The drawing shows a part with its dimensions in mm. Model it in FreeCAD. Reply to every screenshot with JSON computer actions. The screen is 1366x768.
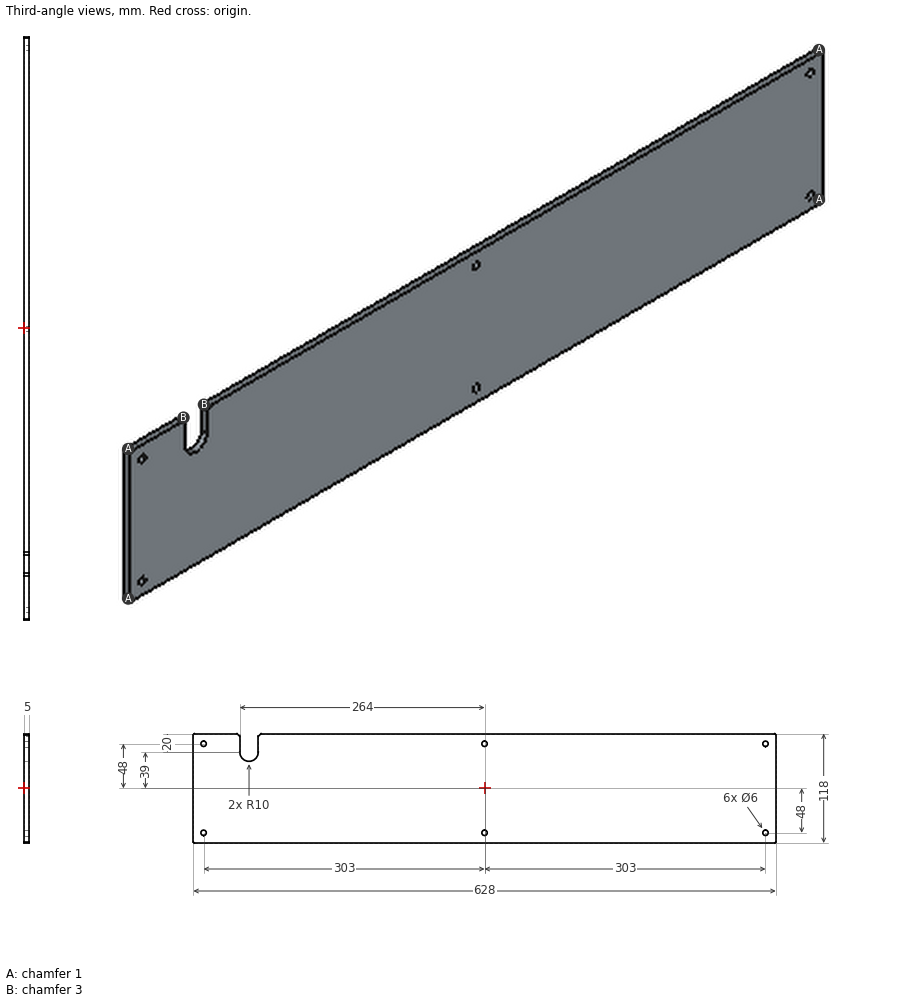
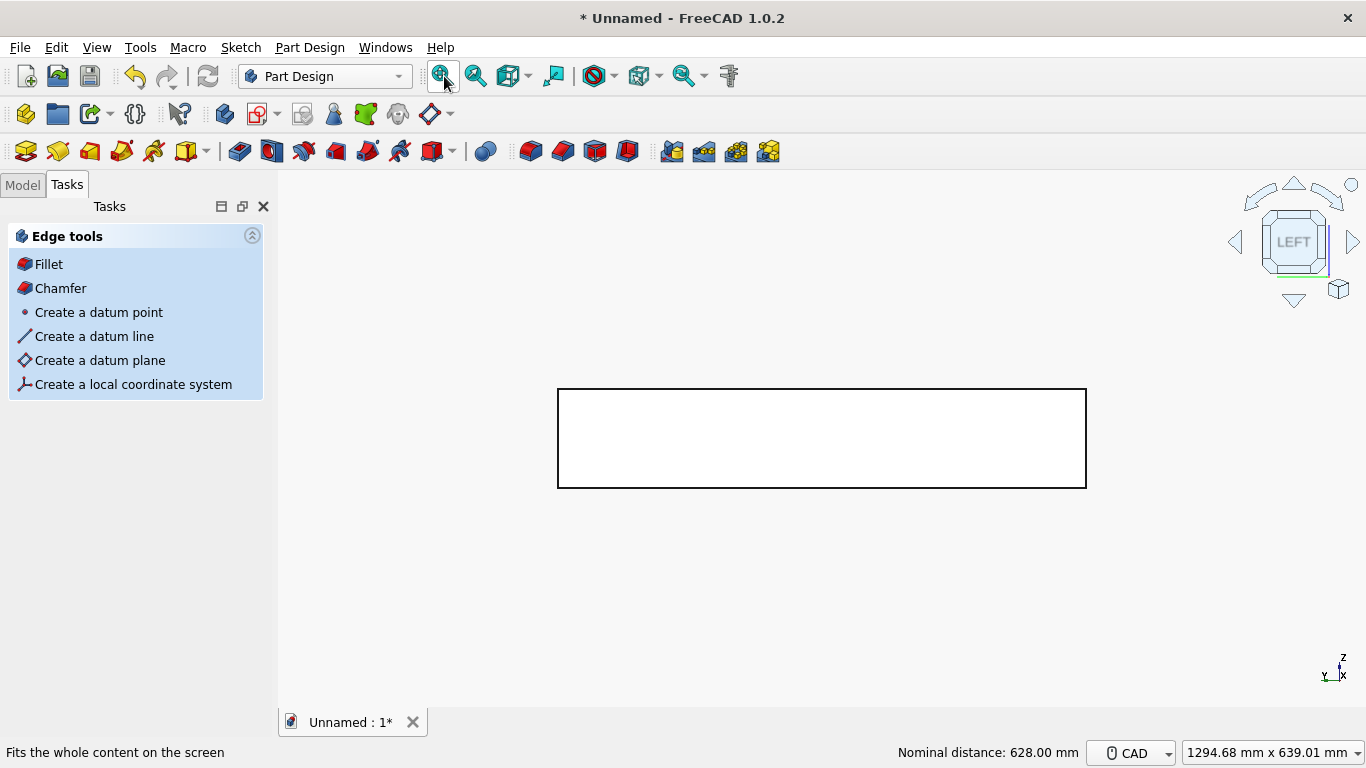
{"action": "key", "text": "v 3"}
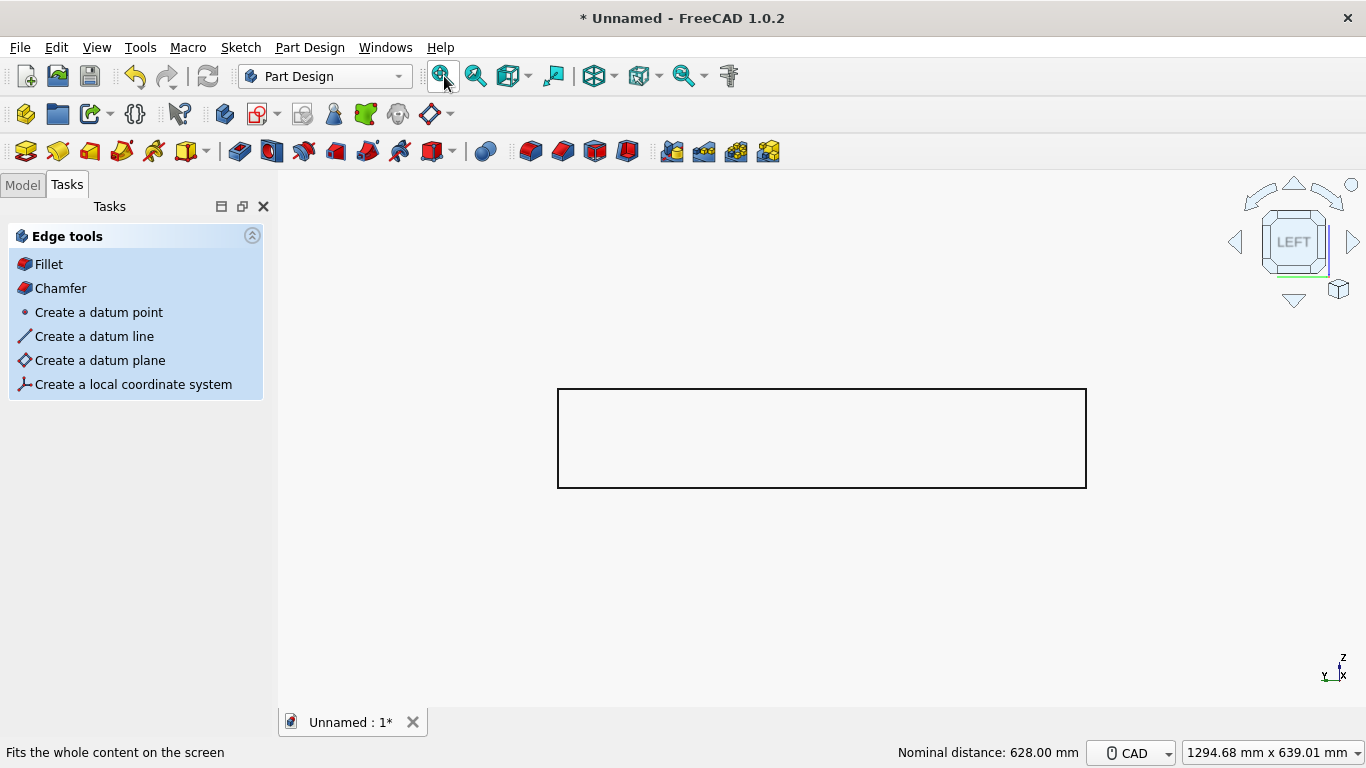
{"action": "key", "text": "0"}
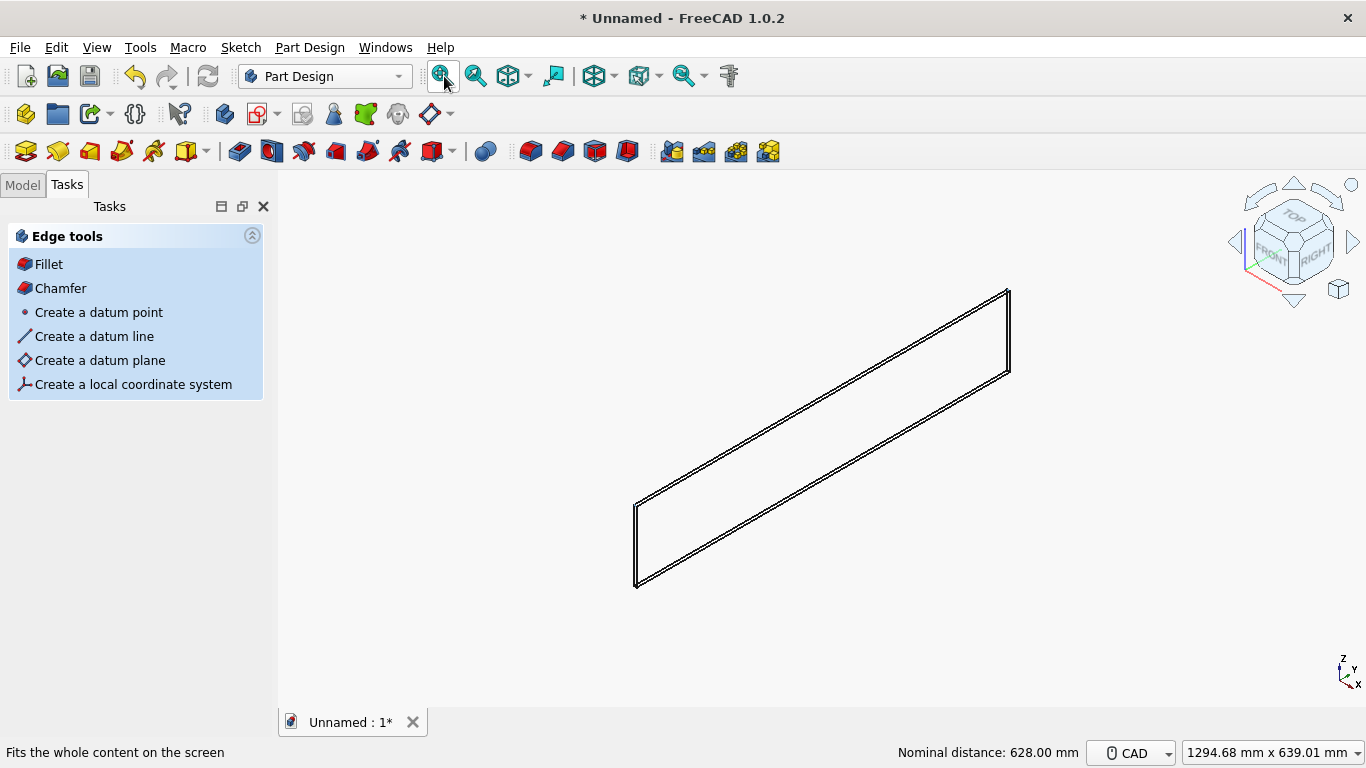
{"action": "scroll", "coordinate": [1009, 370], "scroll_direction": "up", "scroll_amount": 12}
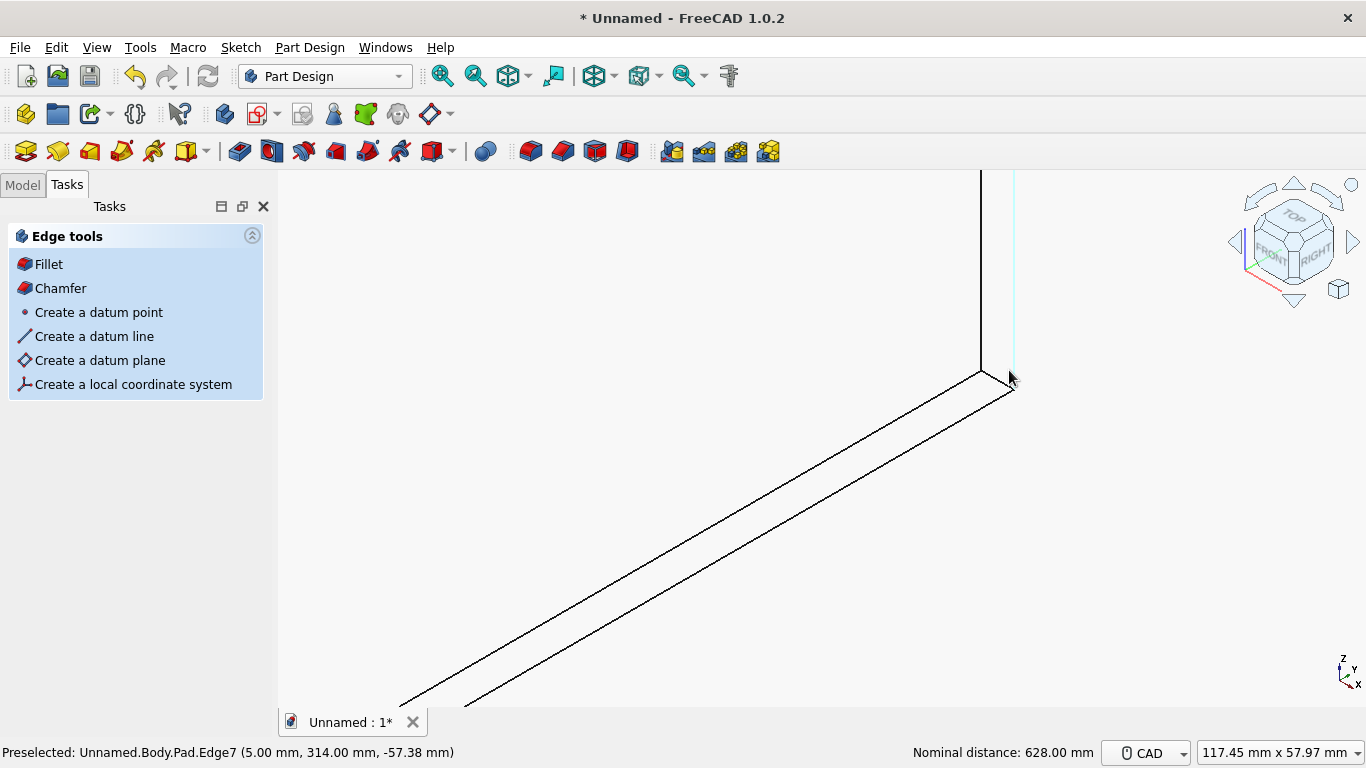
{"action": "left_click", "coordinate": [998, 379], "text": "ctrl"}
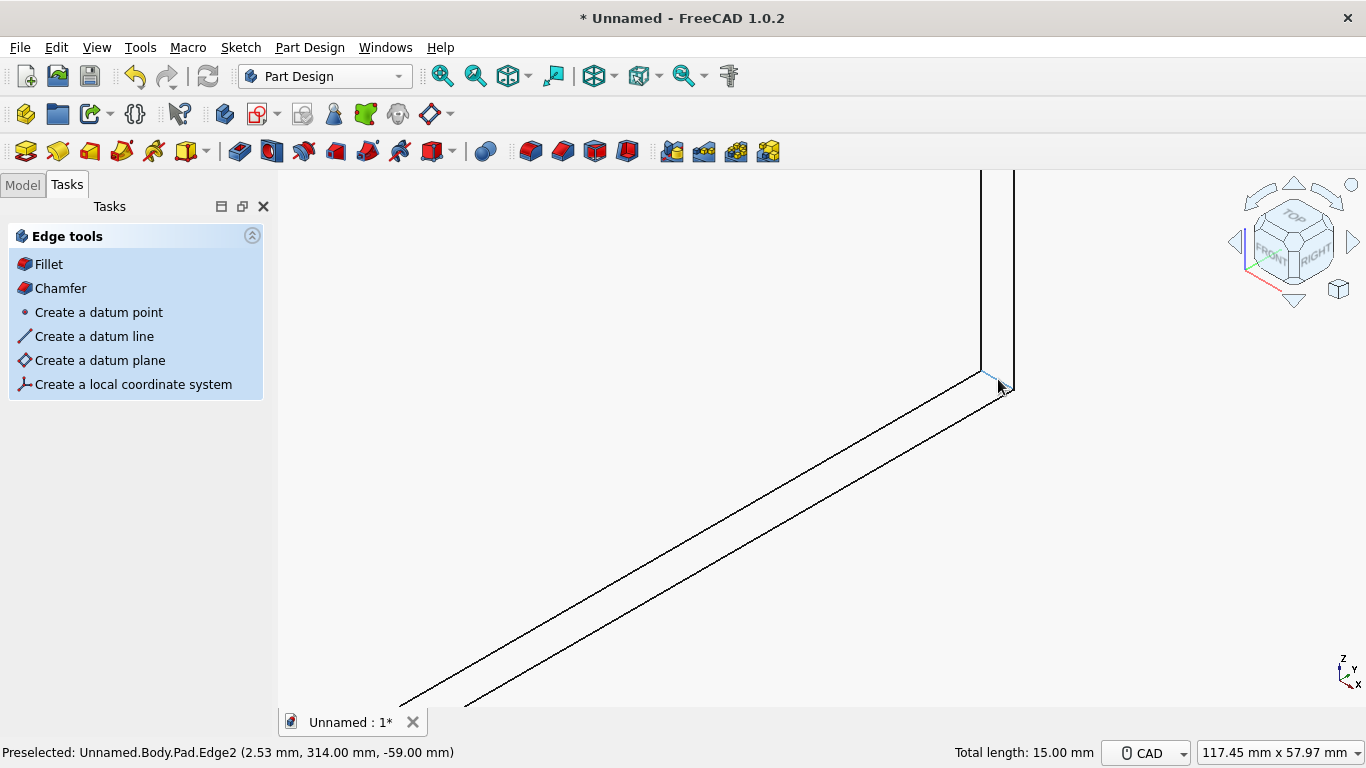
{"action": "left_click", "coordinate": [444, 76]}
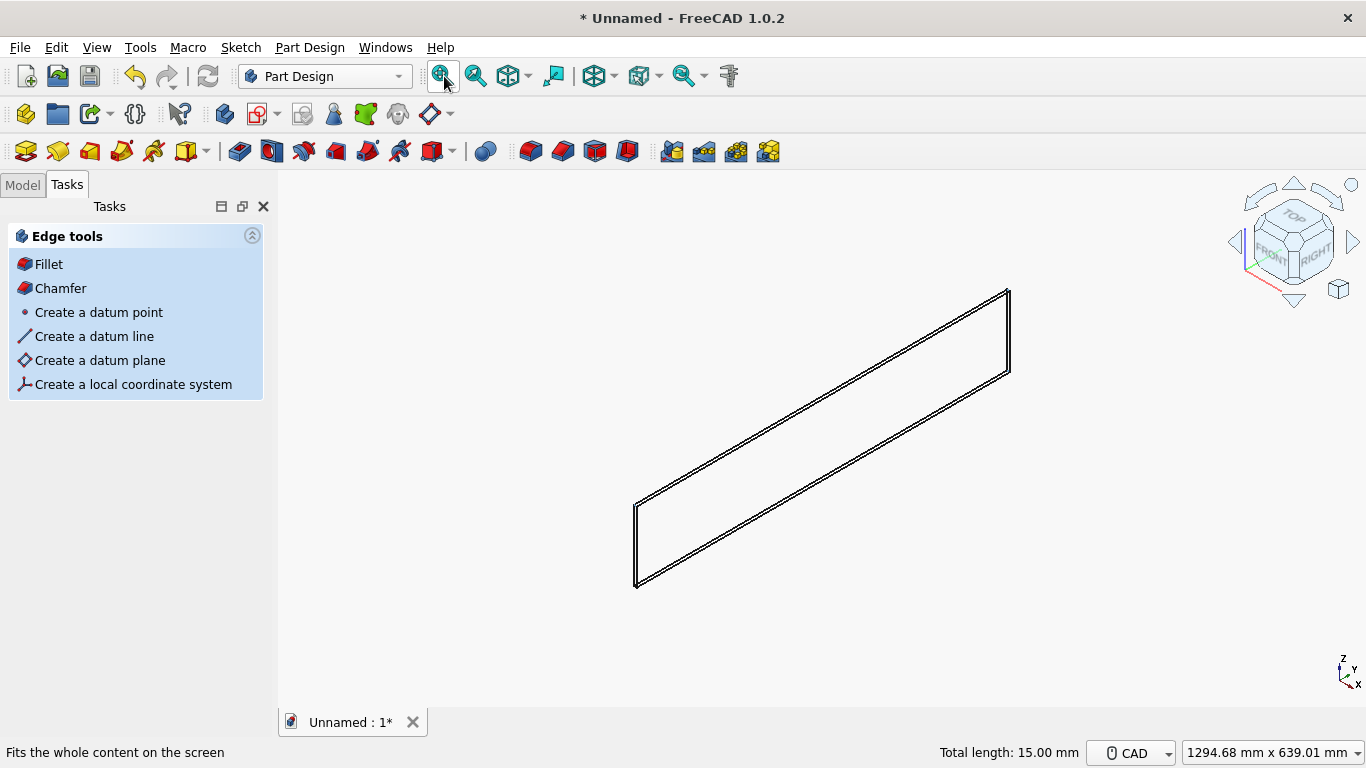
{"action": "key", "text": "2"}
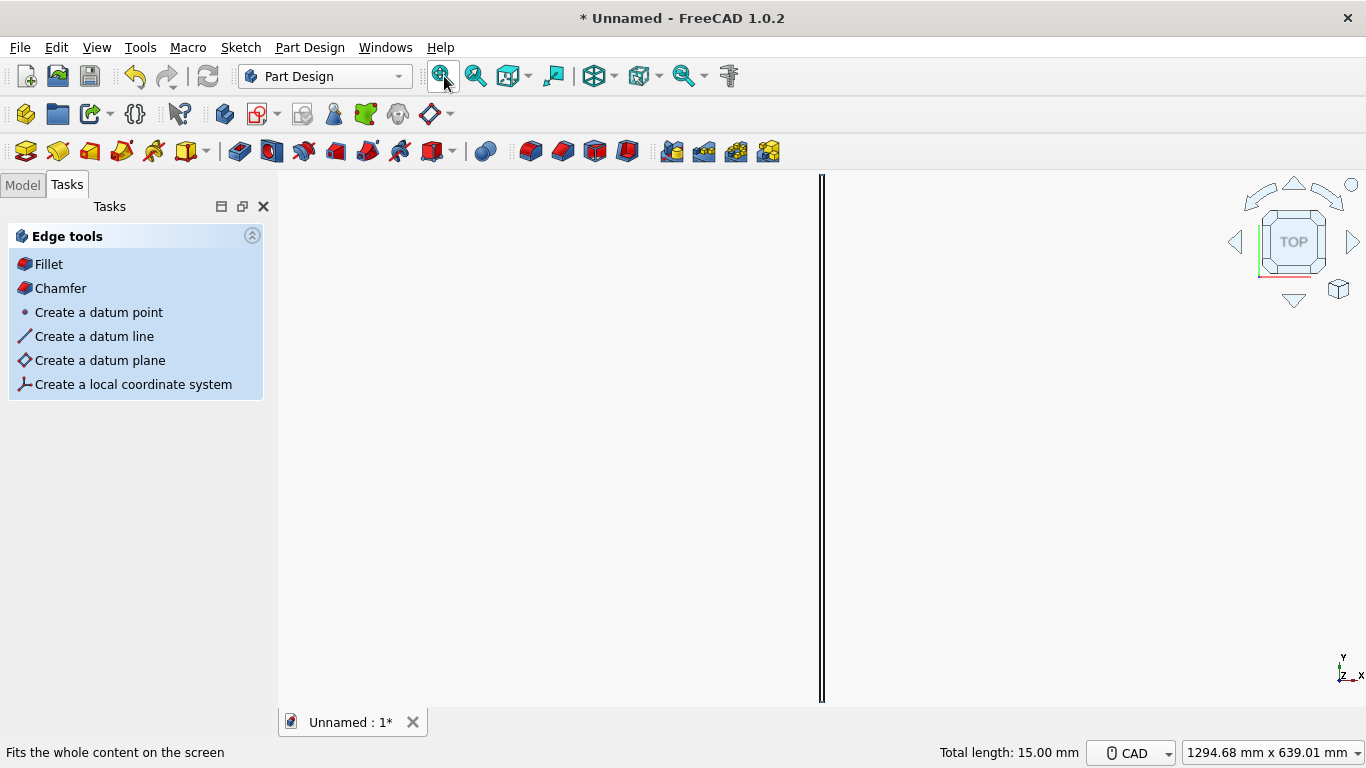
{"action": "key", "text": "1"}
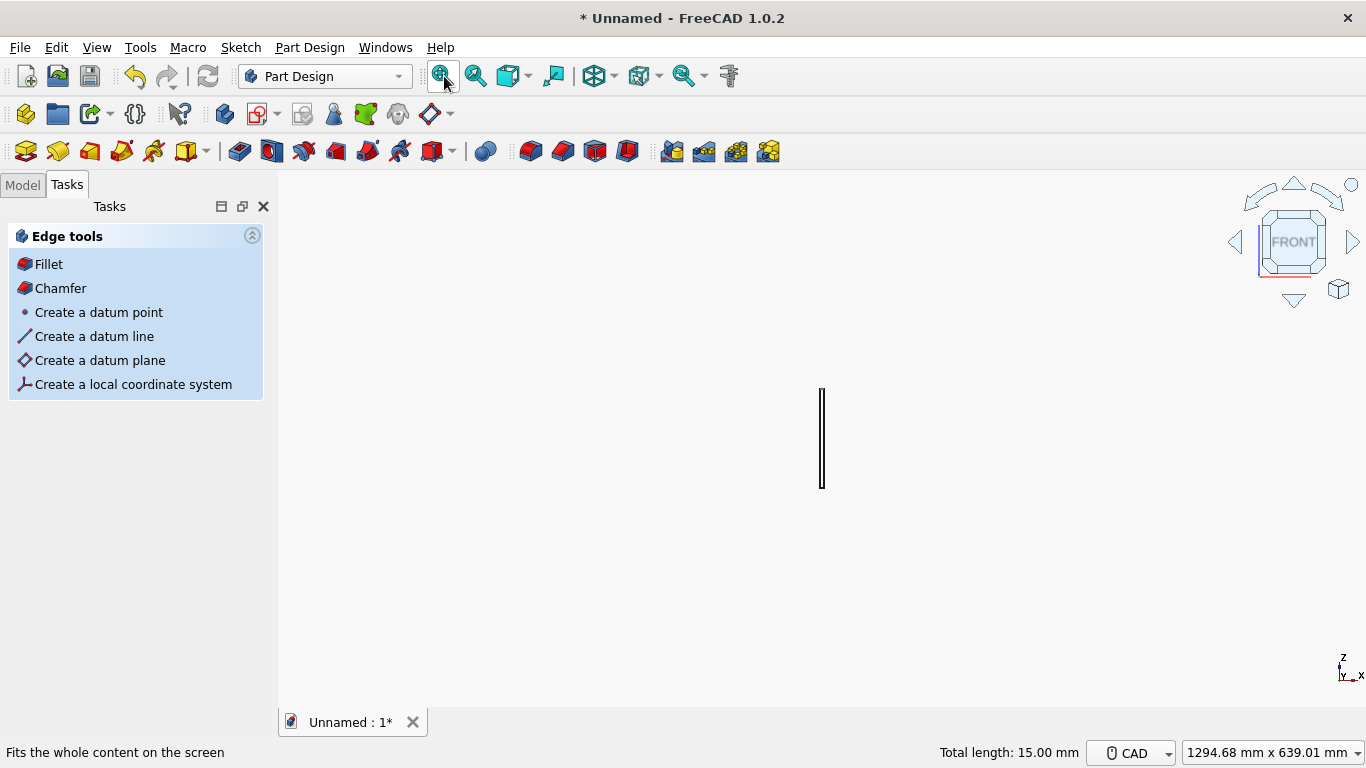
{"action": "key", "text": "v f"}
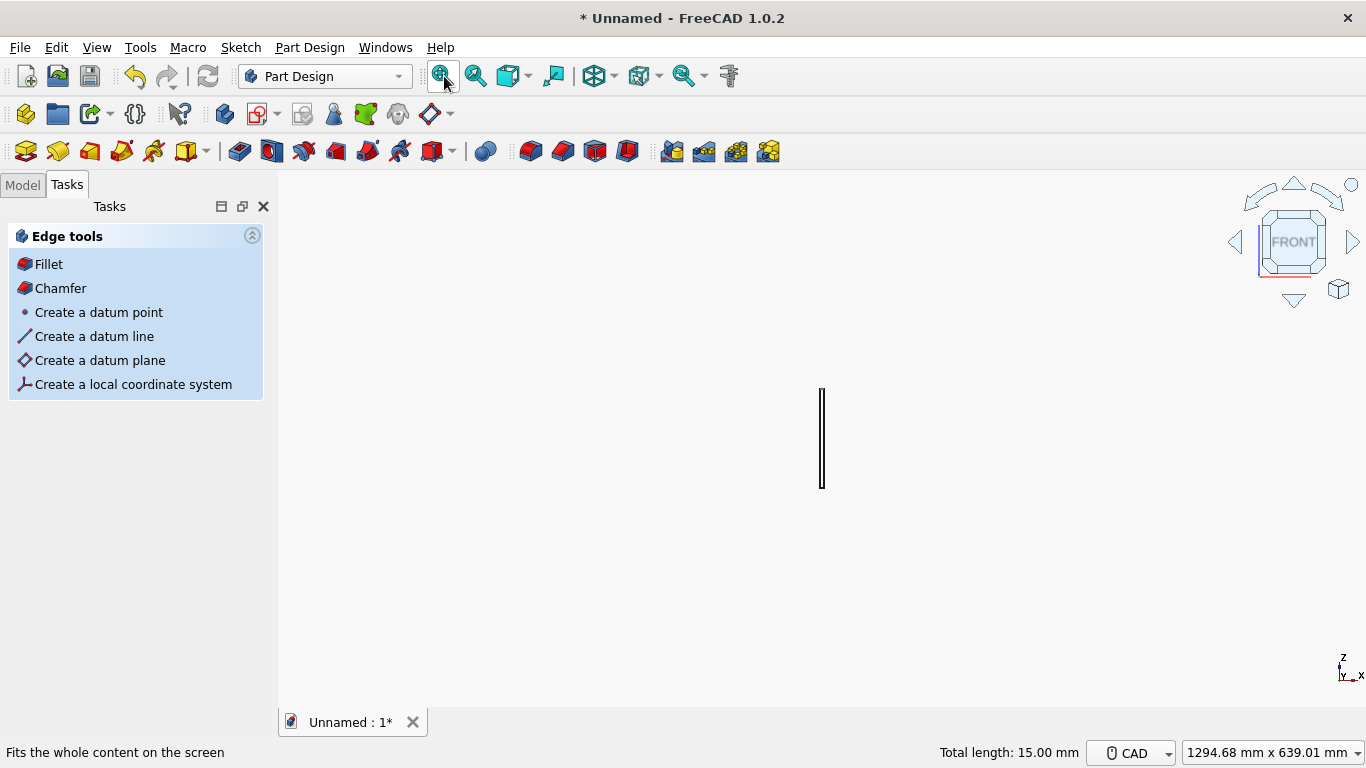
{"action": "left_click", "coordinate": [822, 487], "text": "ctrl"}